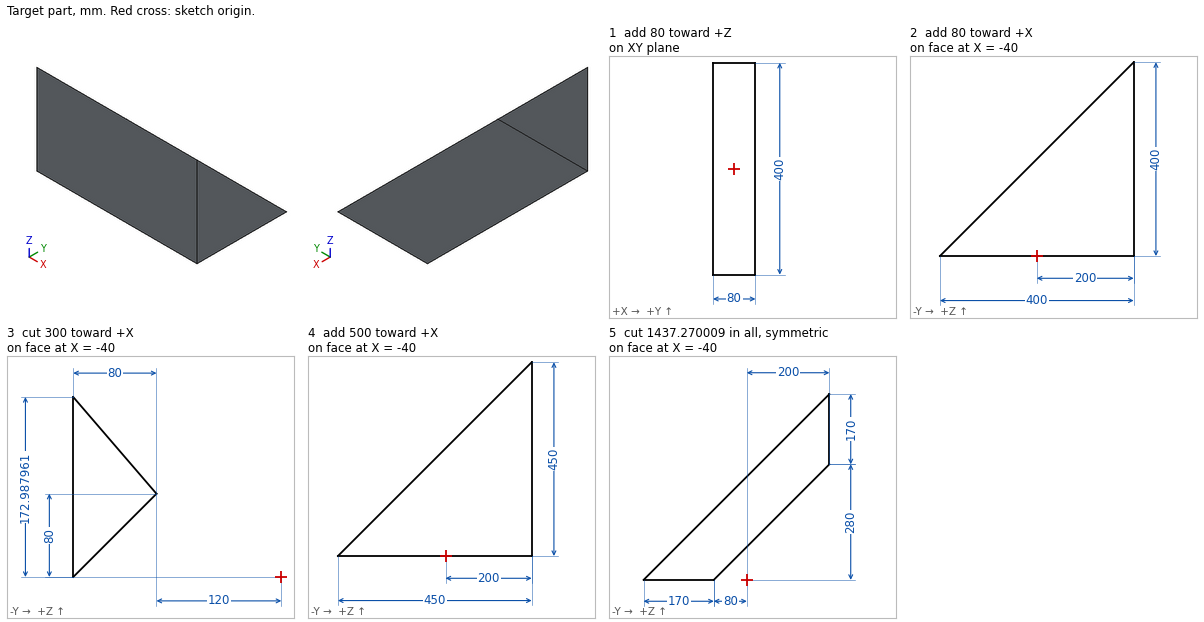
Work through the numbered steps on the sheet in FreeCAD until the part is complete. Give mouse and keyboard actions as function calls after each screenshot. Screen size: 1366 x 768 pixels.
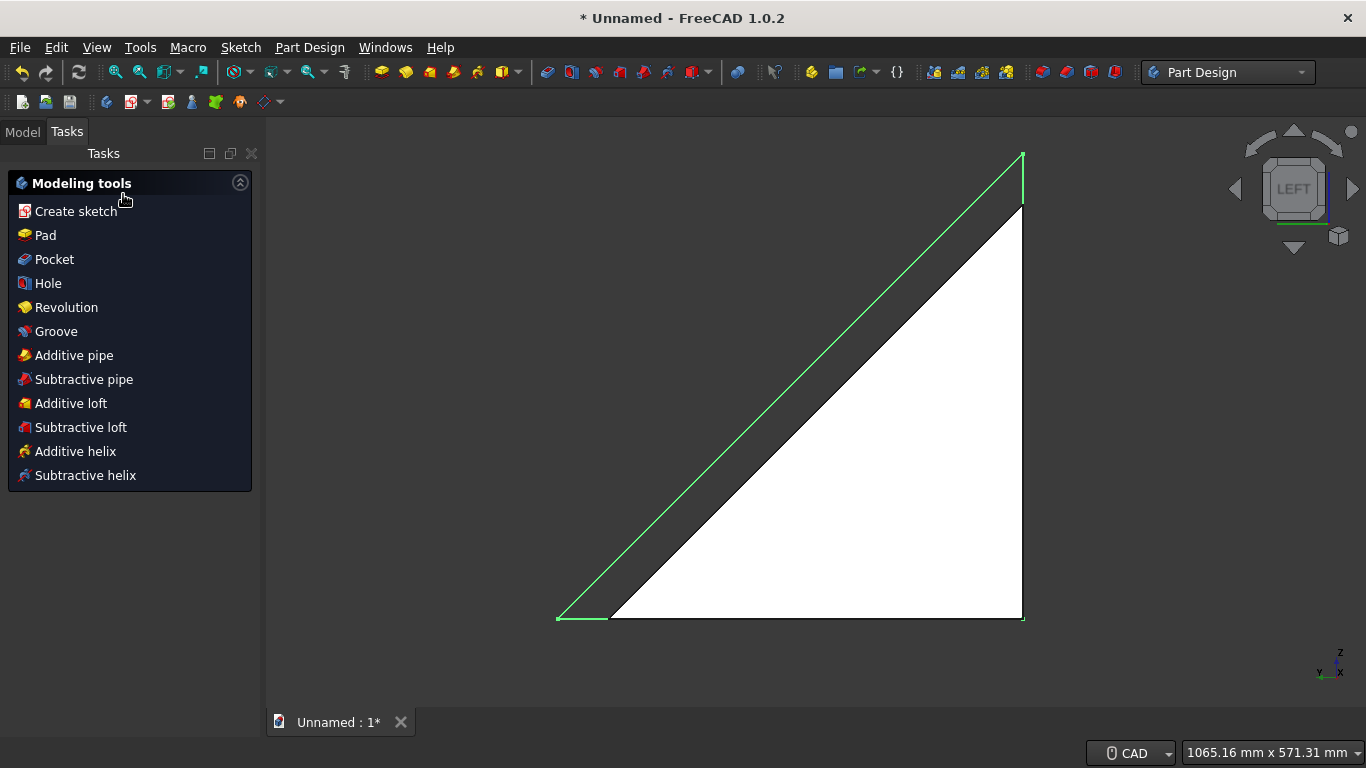
click(382, 72)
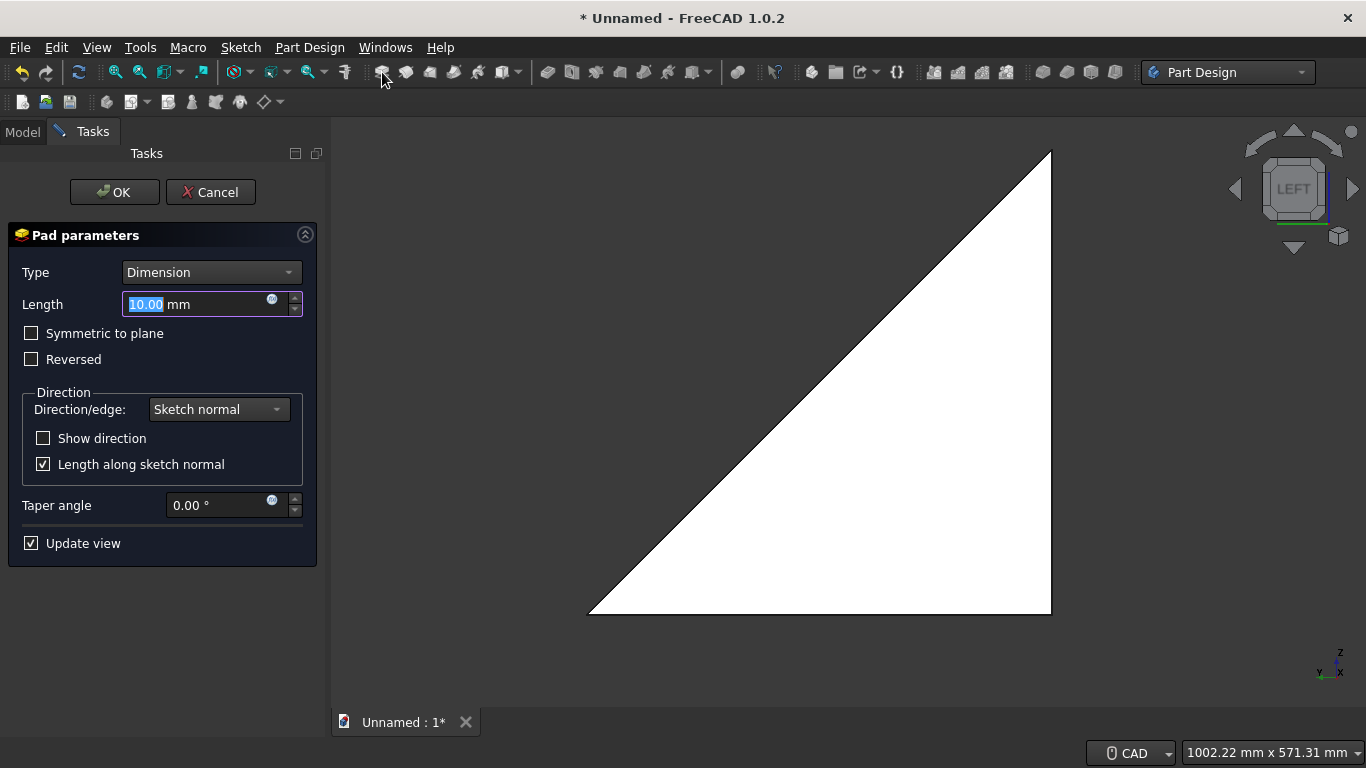
text(500)
key(Tab)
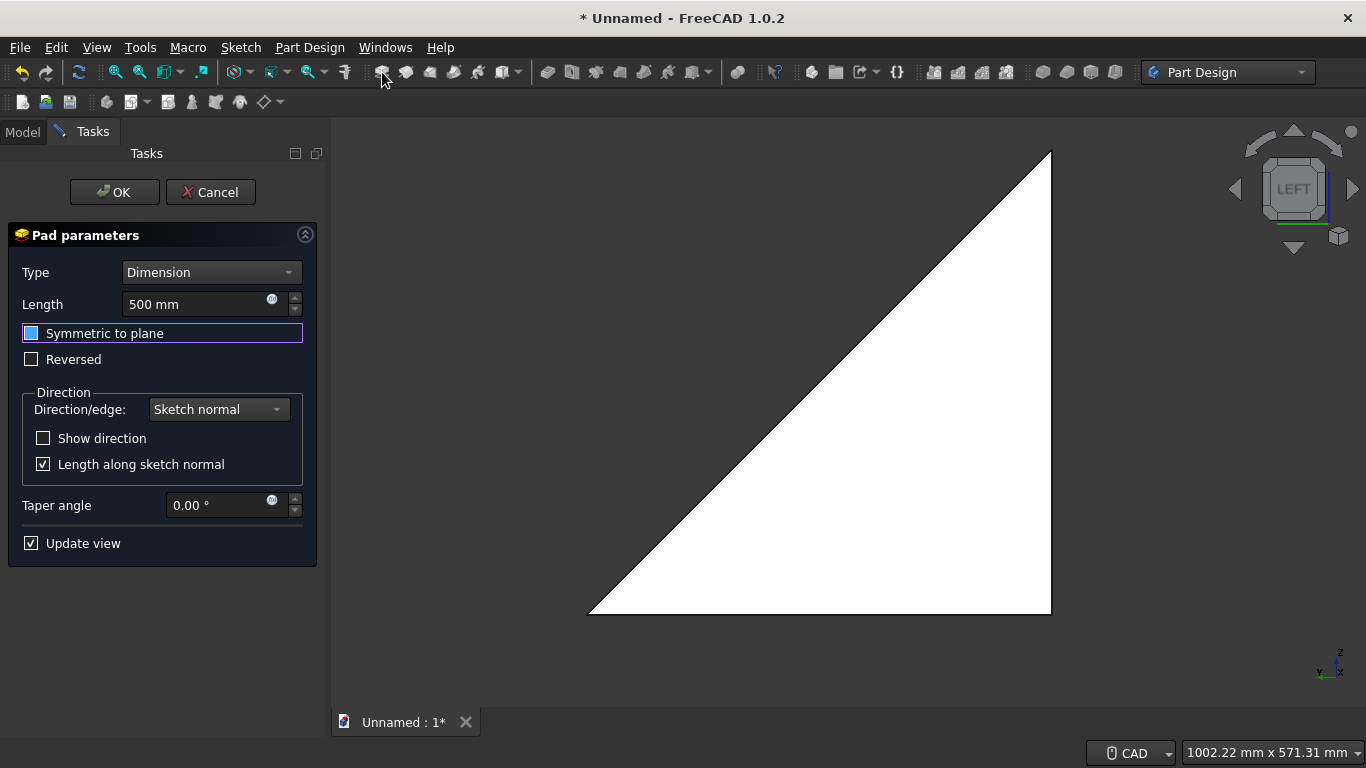
click(30, 359)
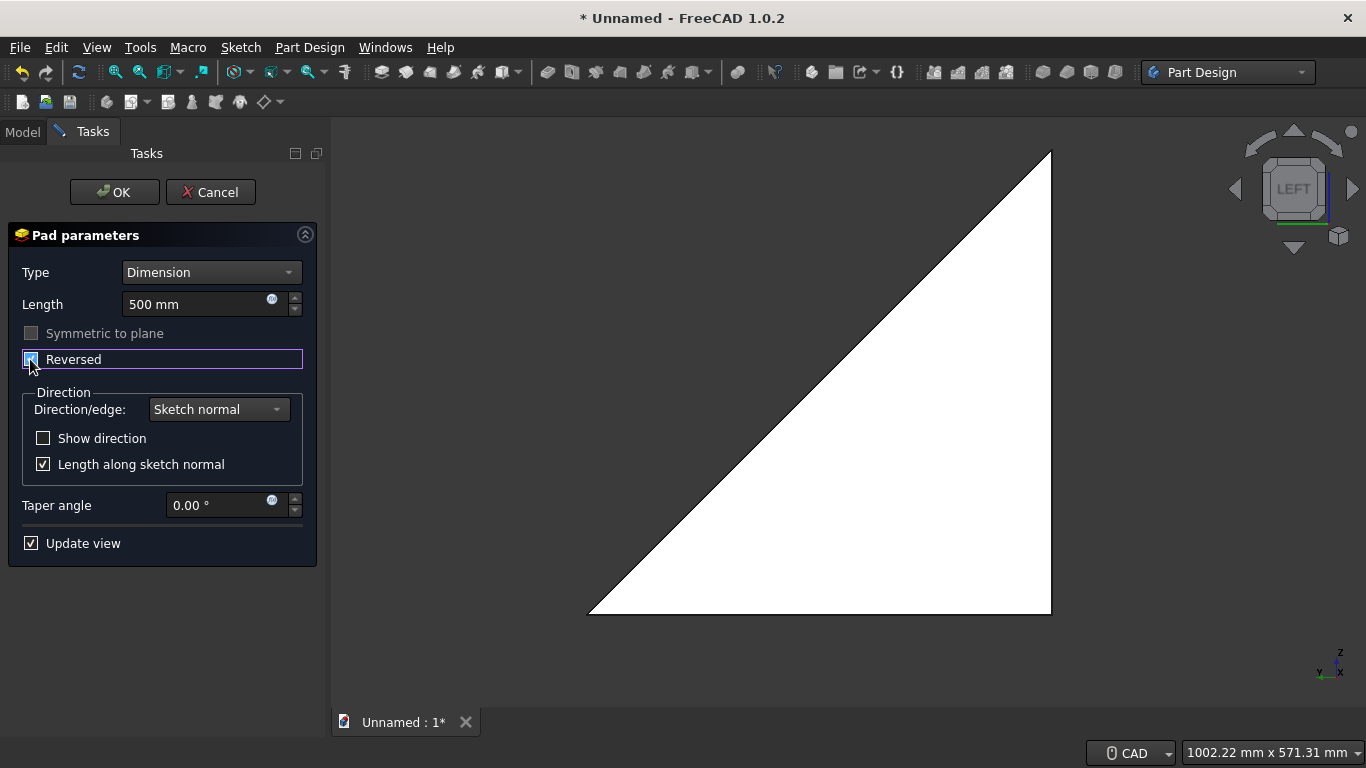
click(115, 192)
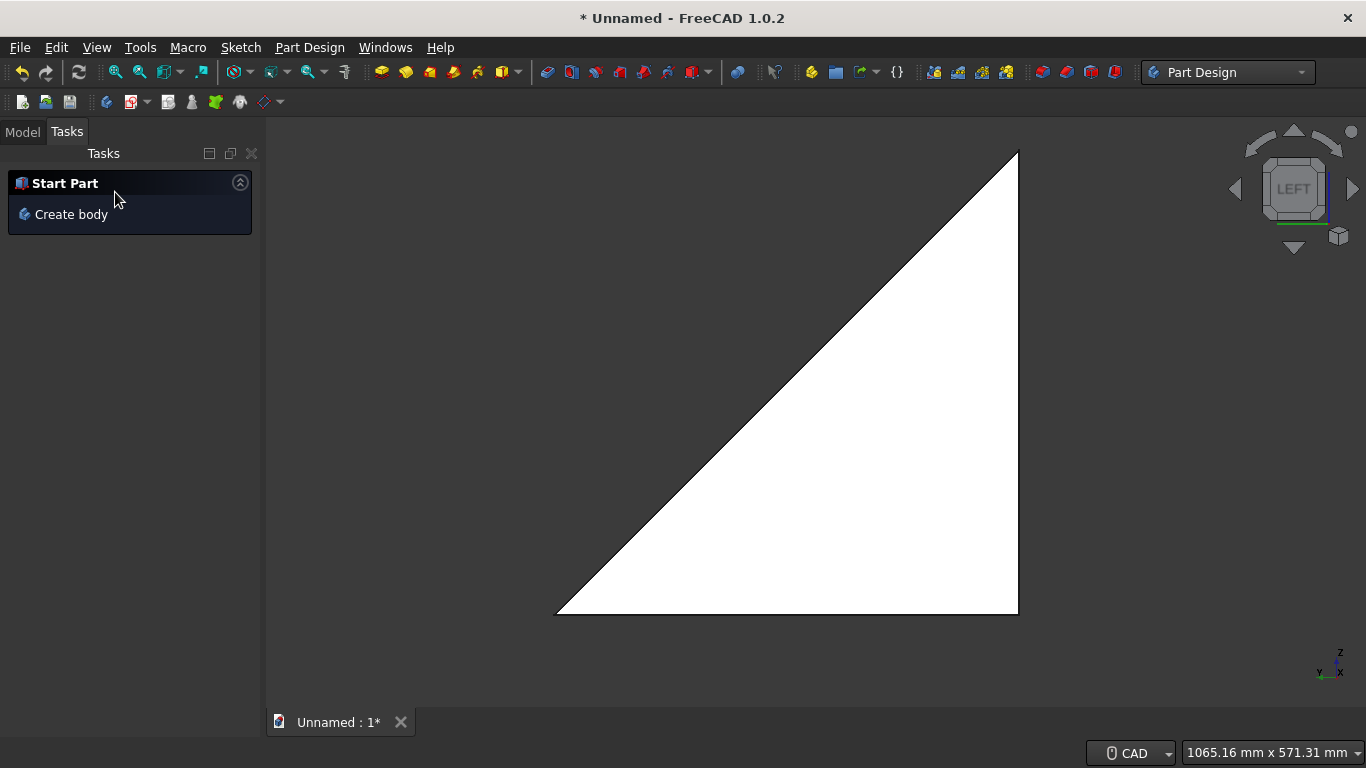
click(919, 448)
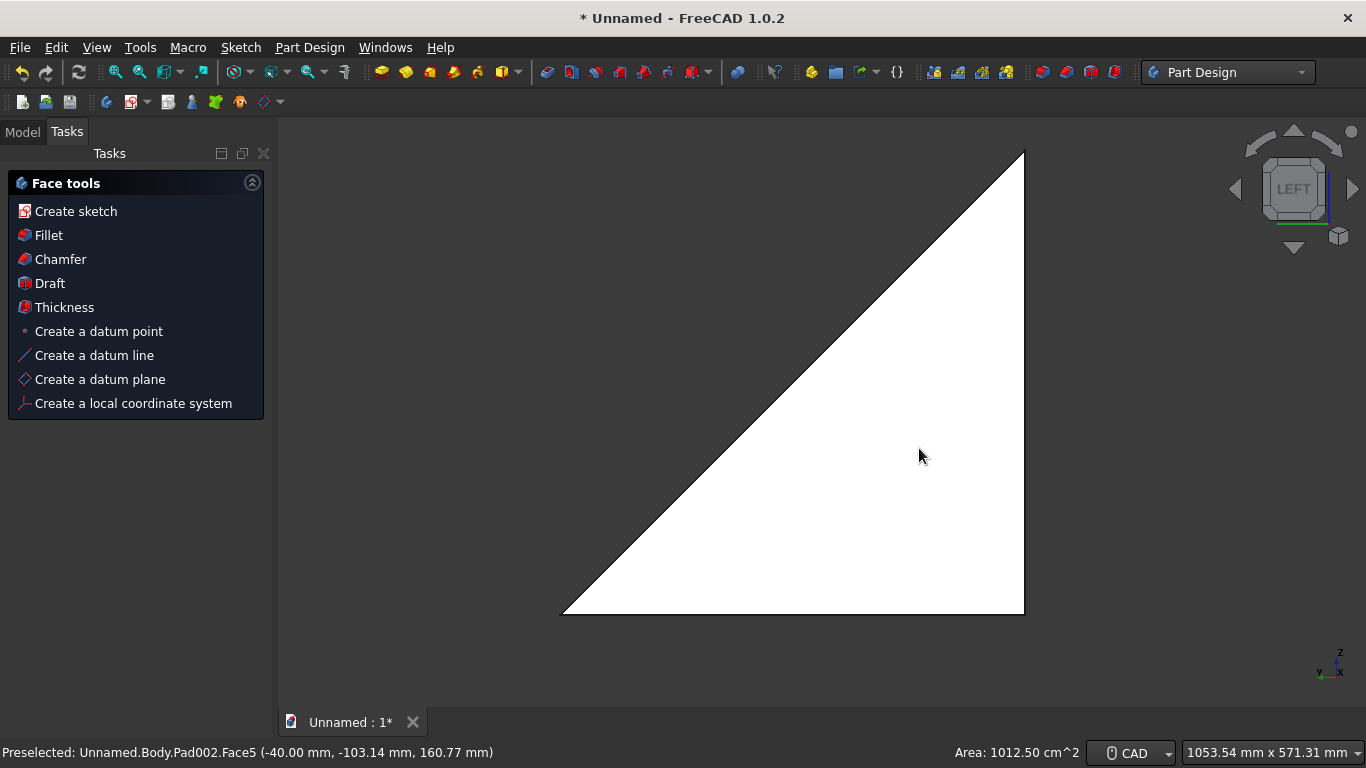
click(132, 102)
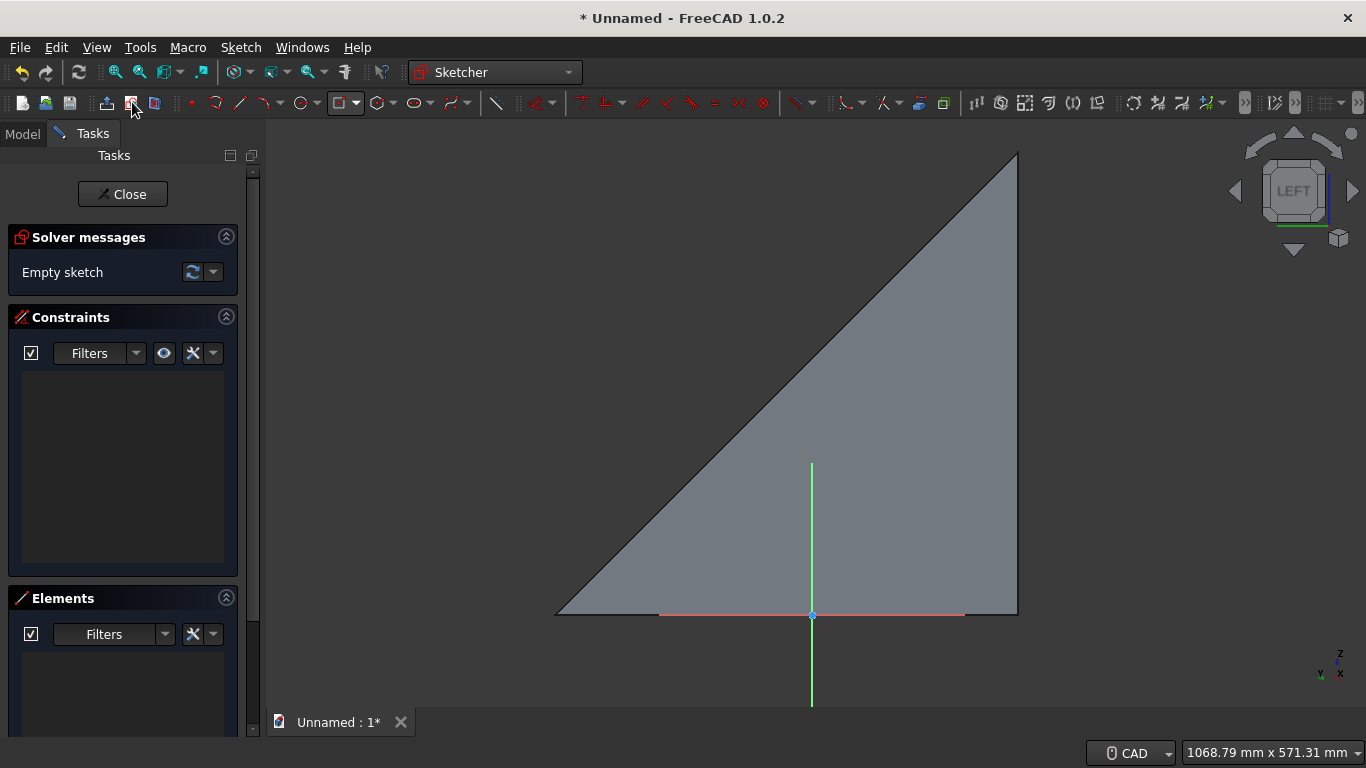
scroll(570, 545, down, 1)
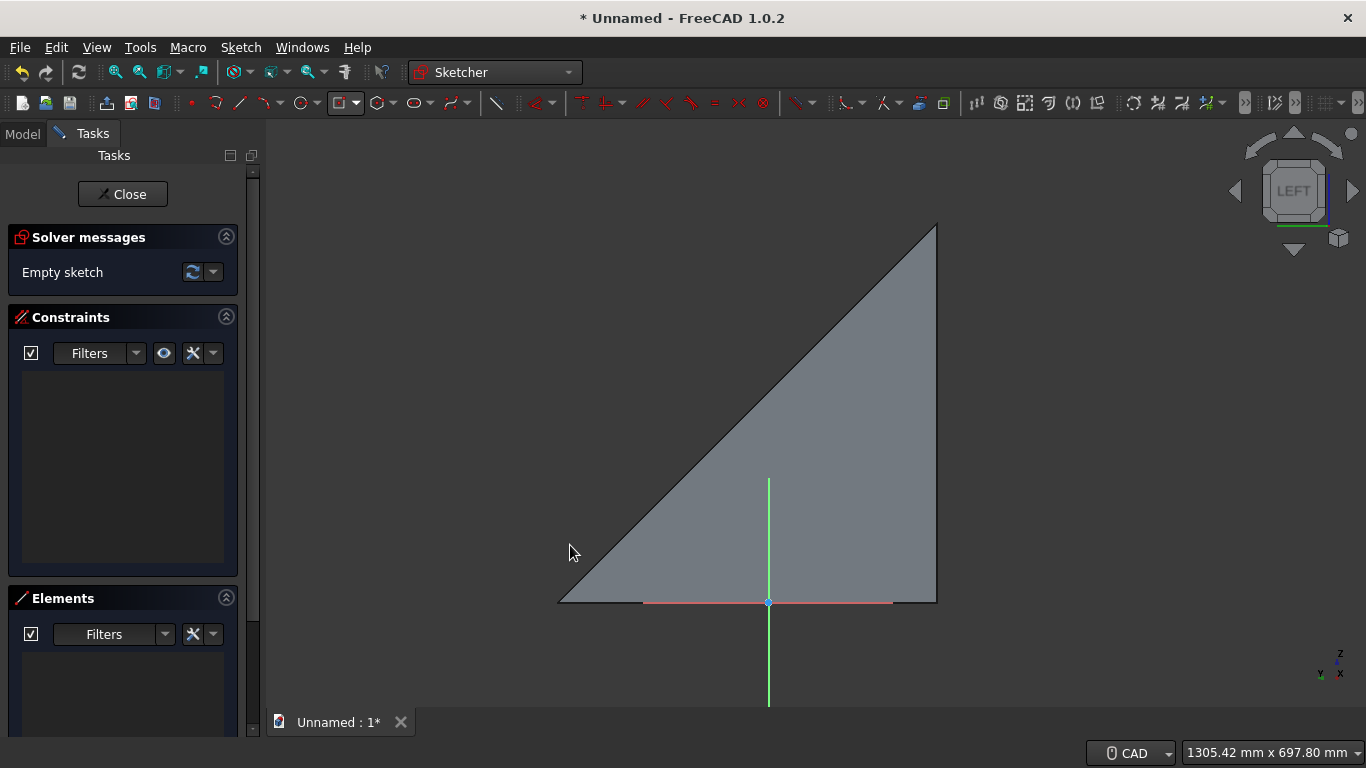
click(216, 104)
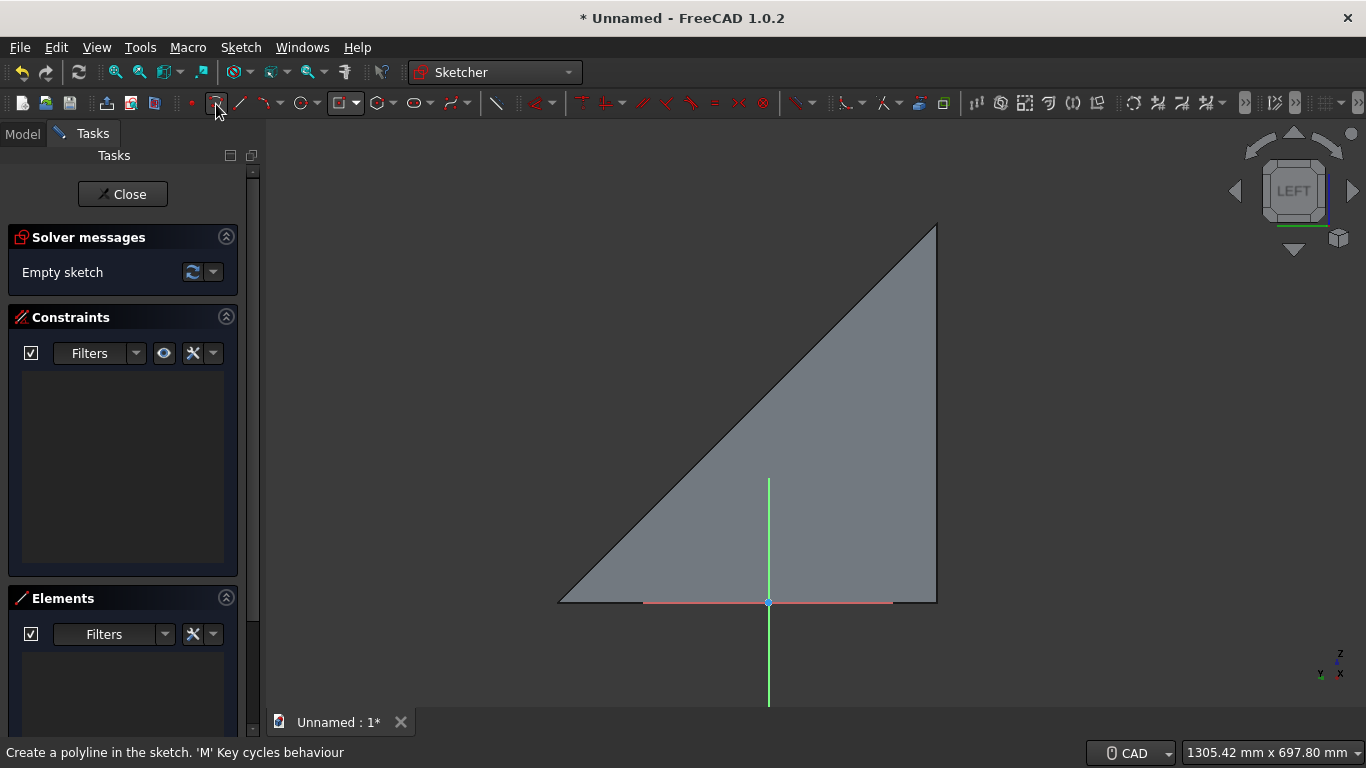
click(701, 603)
click(937, 367)
click(937, 224)
click(558, 594)
click(701, 603)
key(Escape)
key(Escape)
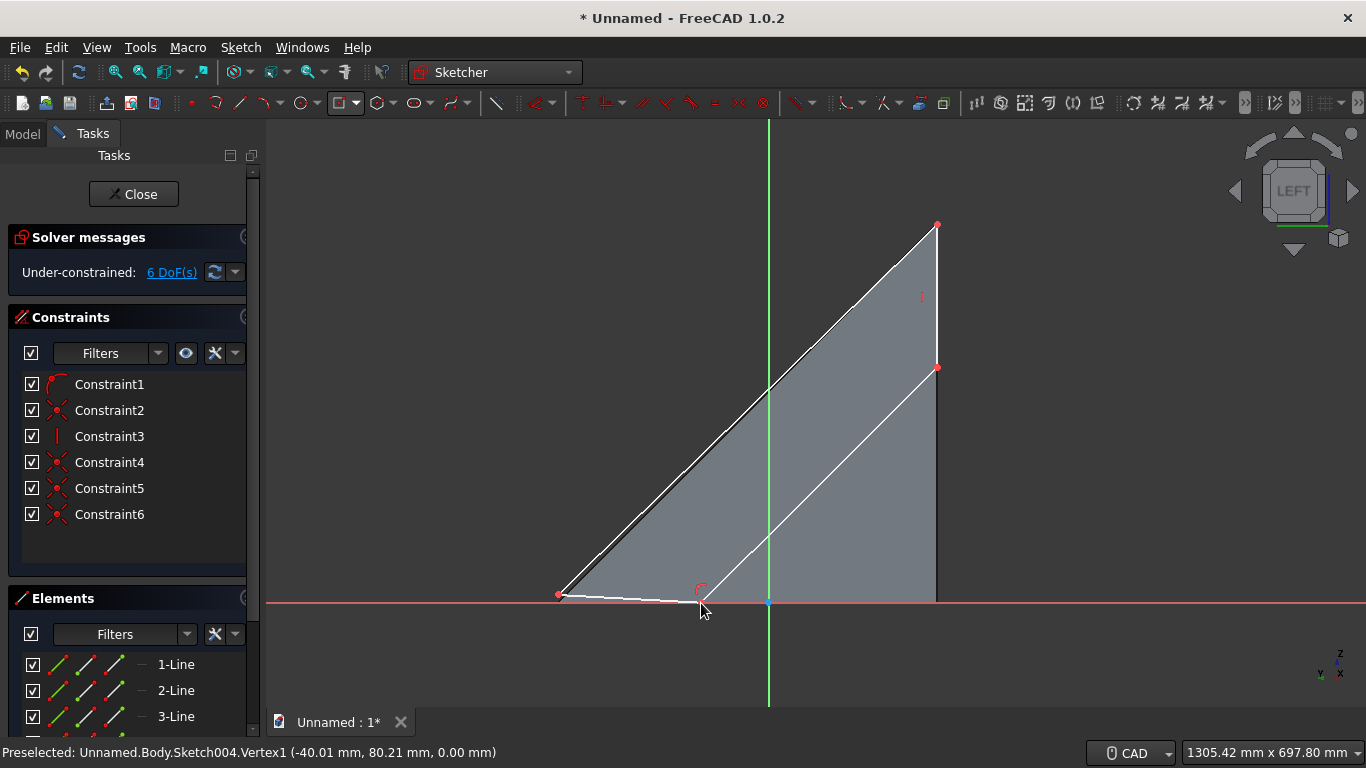
click(658, 600)